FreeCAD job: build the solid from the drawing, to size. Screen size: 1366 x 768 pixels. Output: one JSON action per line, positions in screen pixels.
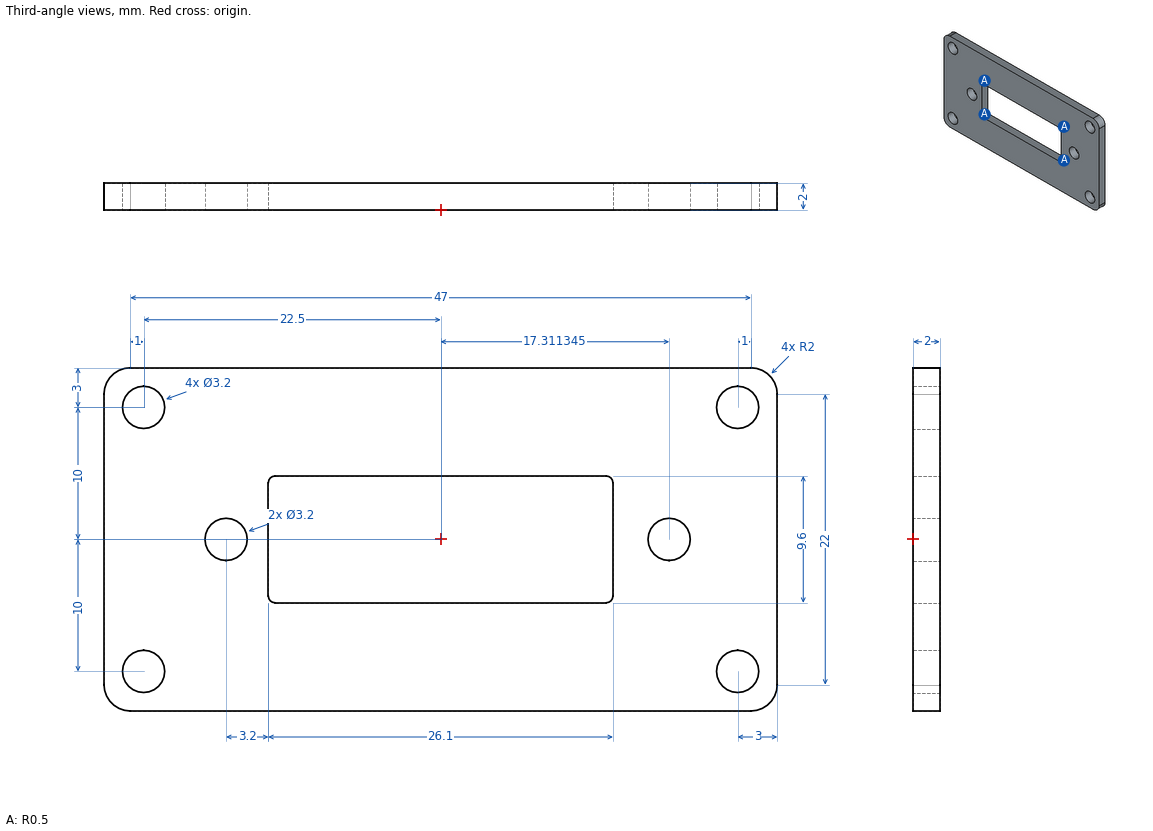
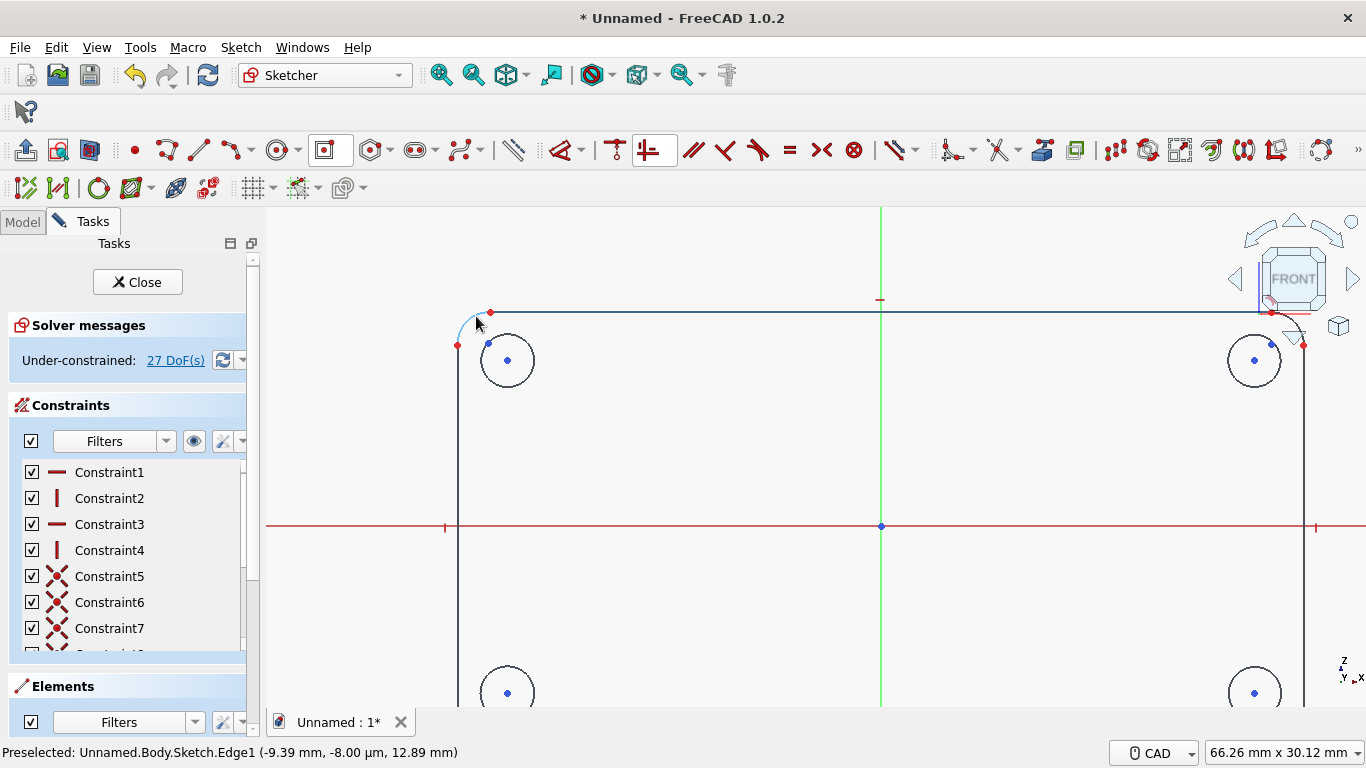
{"action": "left_click", "coordinate": [475, 315]}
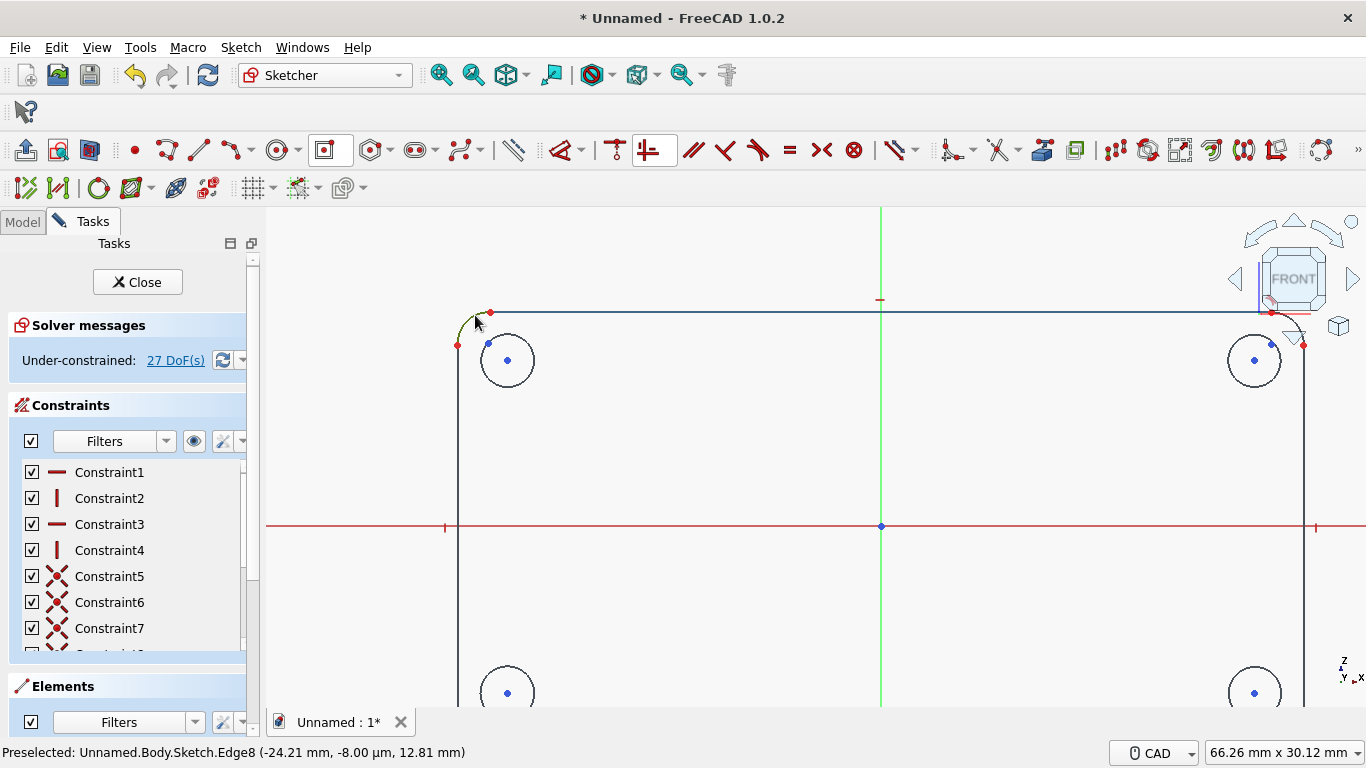
{"action": "left_click", "coordinate": [758, 150]}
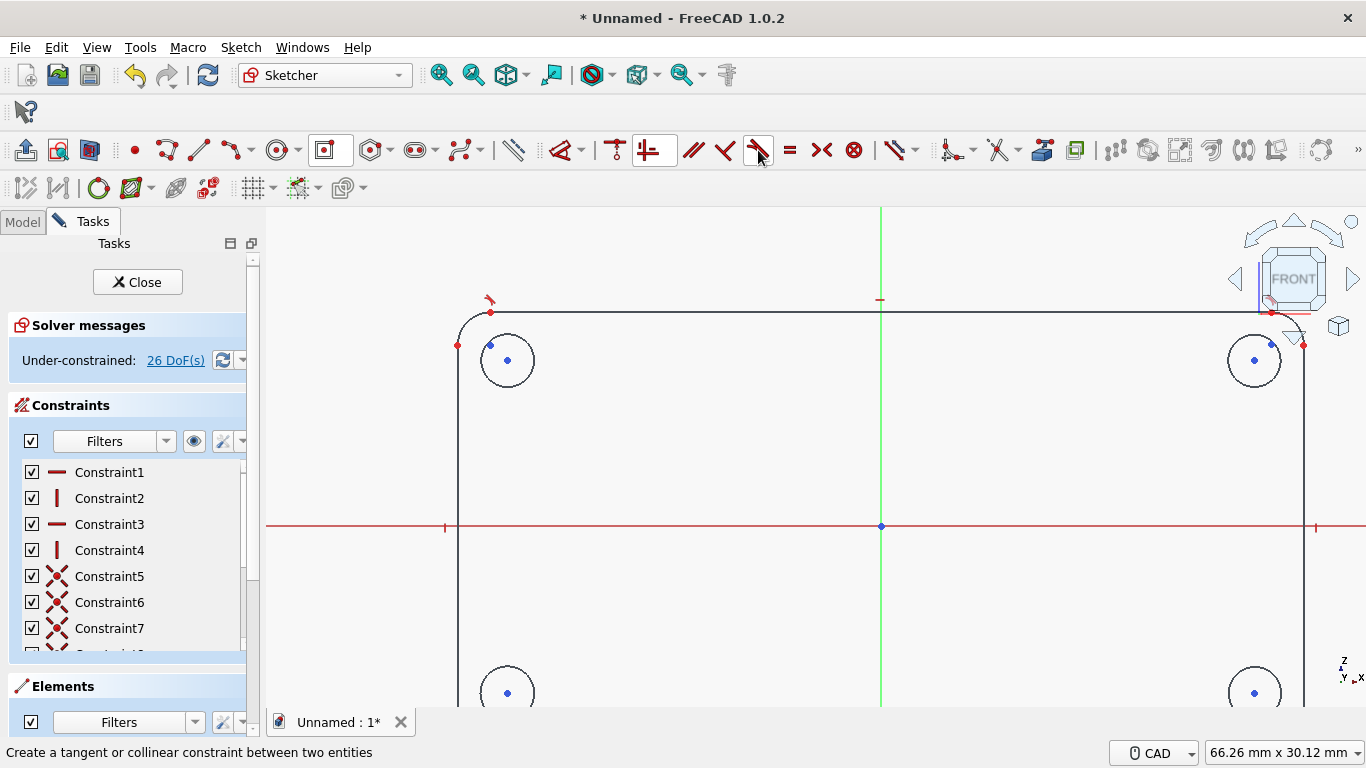
{"action": "scroll", "coordinate": [476, 316], "scroll_direction": "down", "scroll_amount": 2}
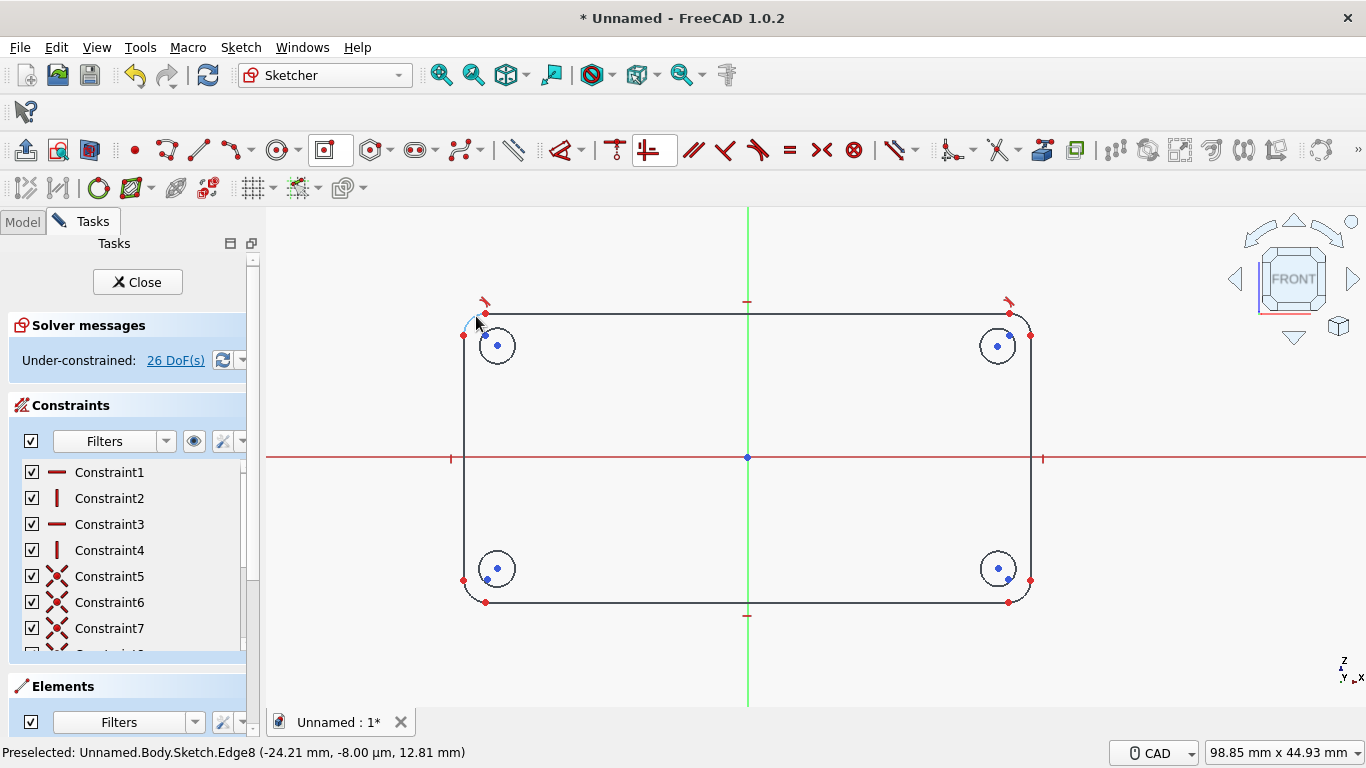
{"action": "left_click", "coordinate": [1031, 409]}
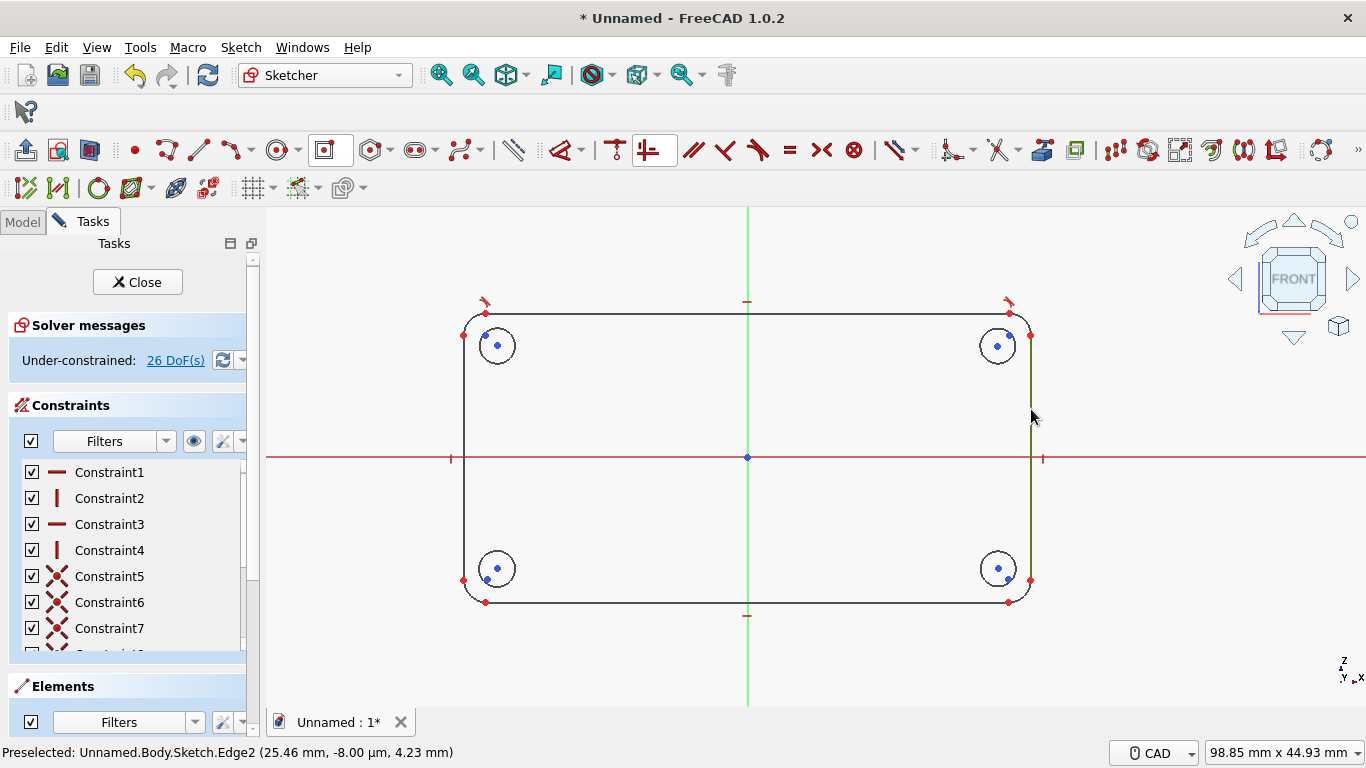
{"action": "scroll", "coordinate": [1029, 326], "scroll_direction": "up", "scroll_amount": 2}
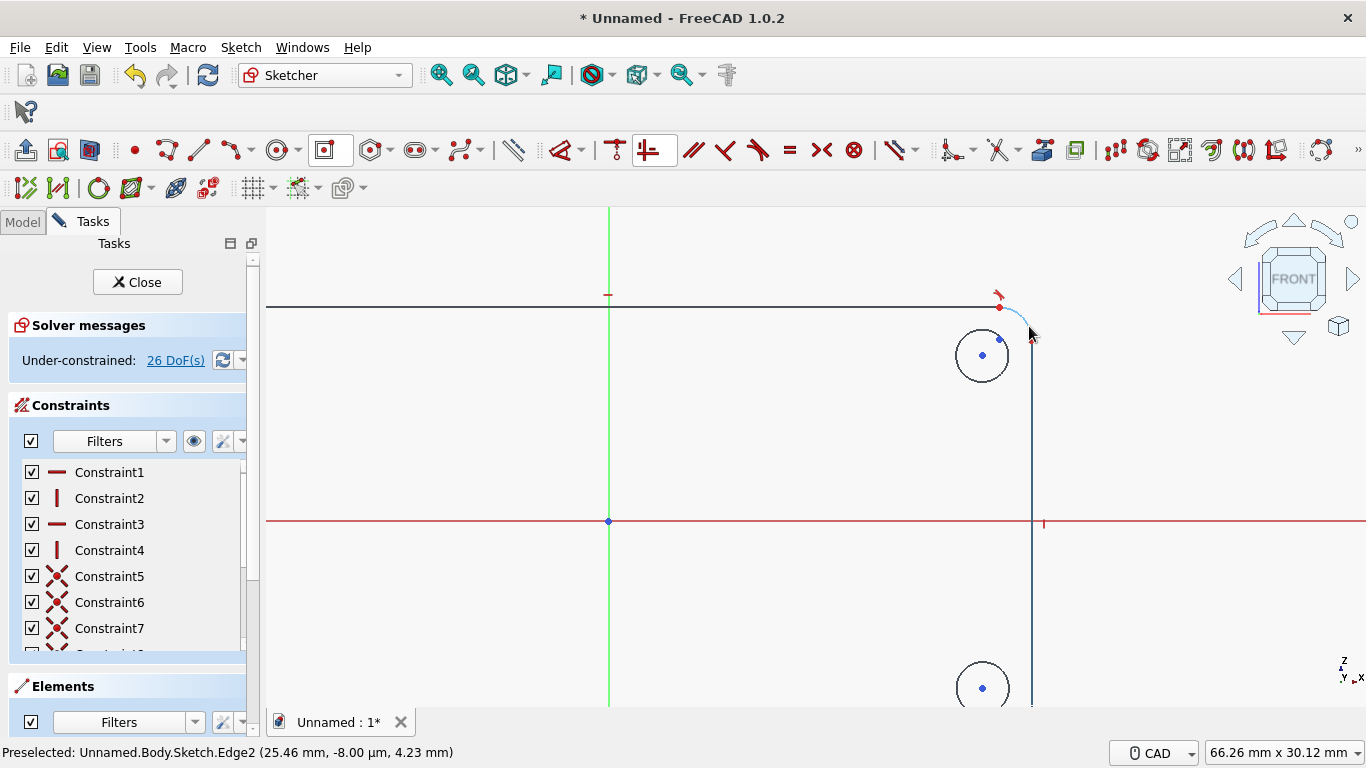
{"action": "left_click", "coordinate": [1028, 325]}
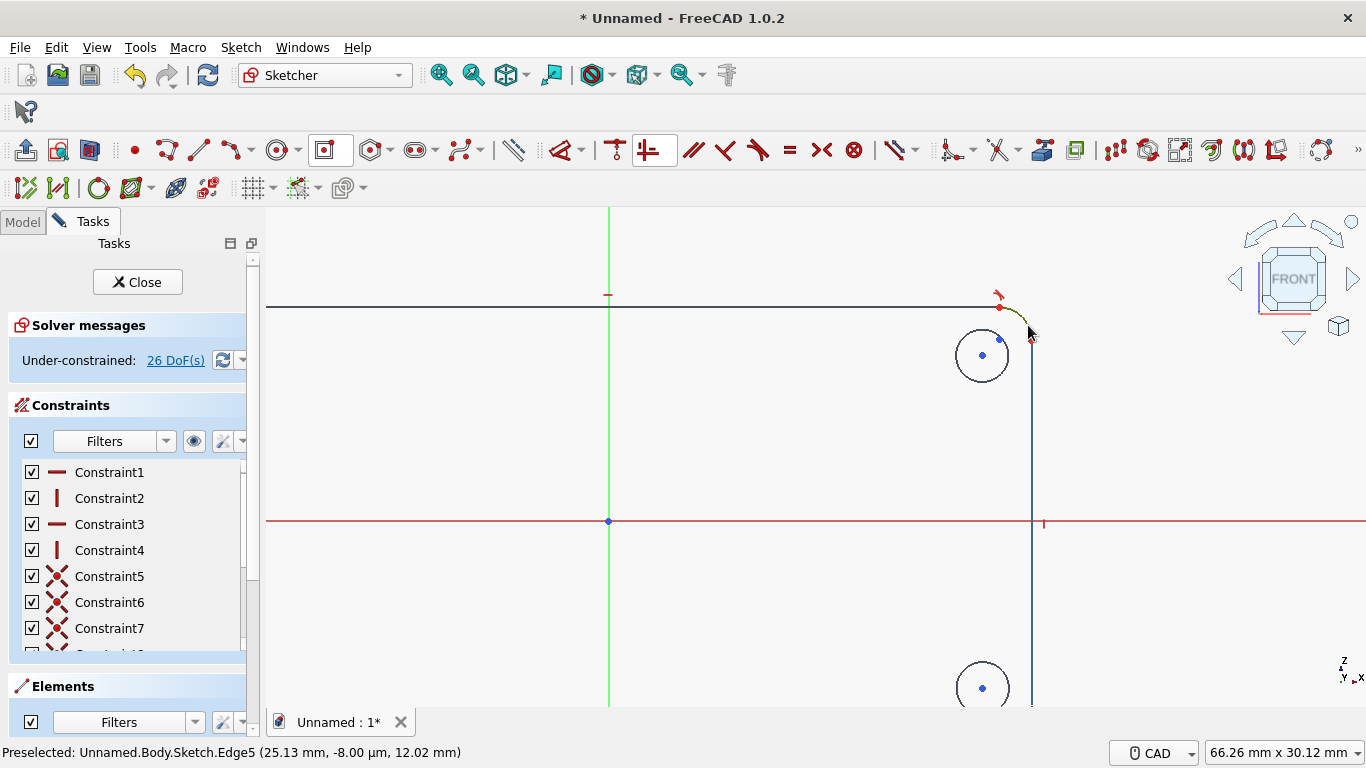
{"action": "left_click", "coordinate": [758, 150]}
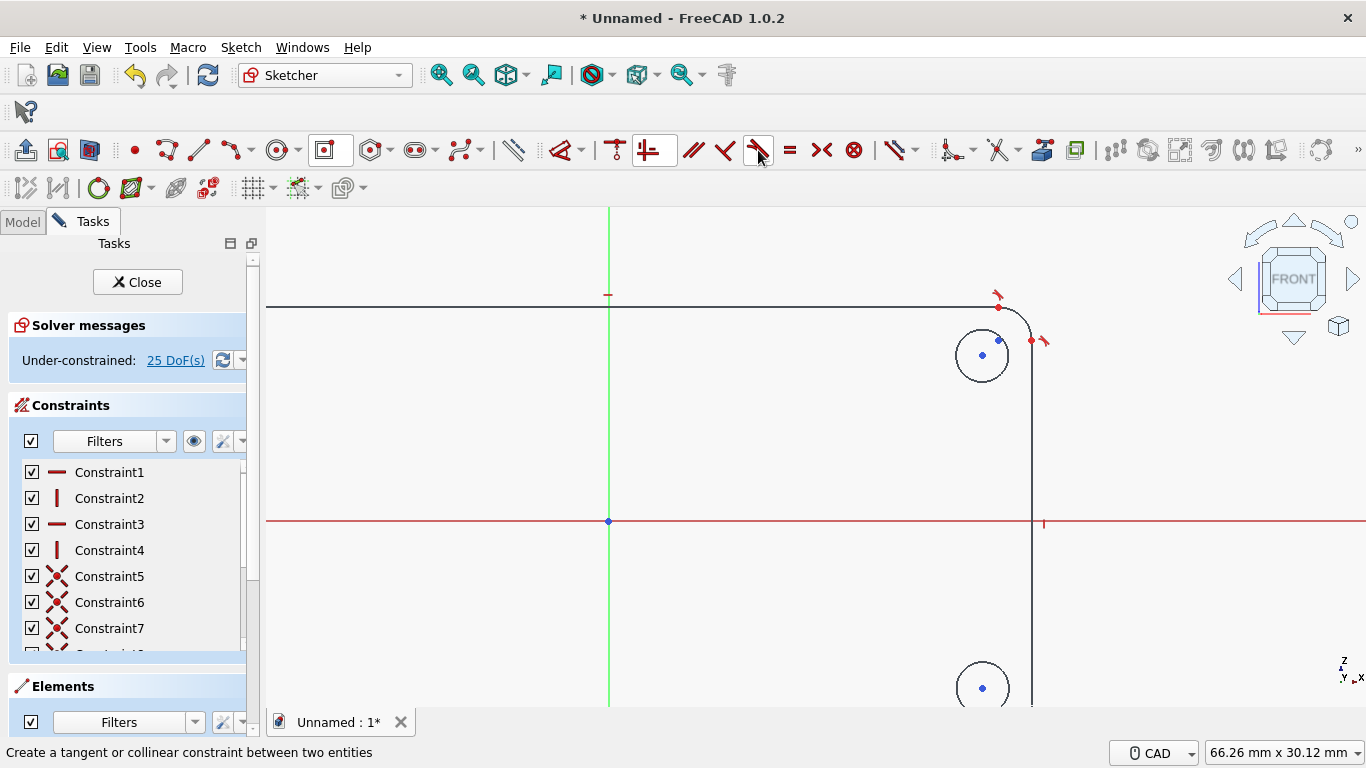
{"action": "left_click", "coordinate": [1032, 450]}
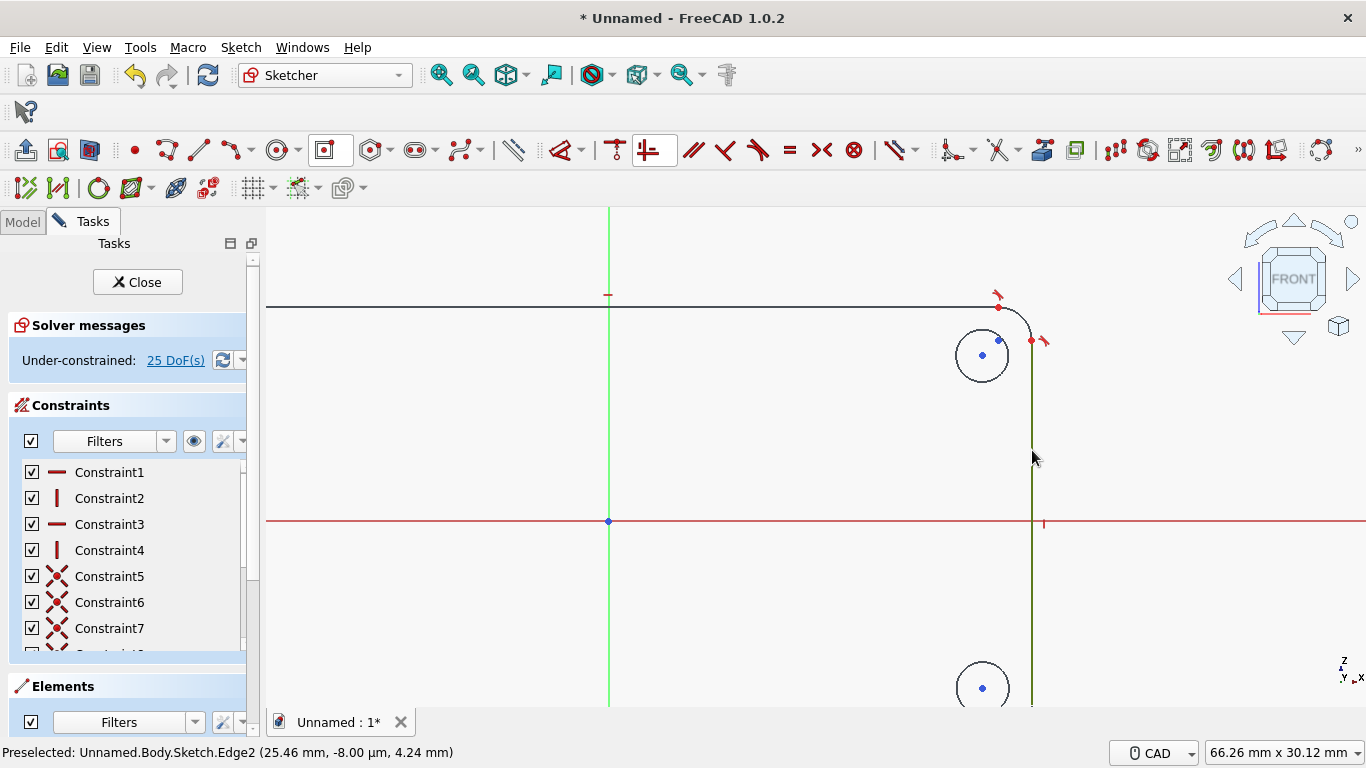
{"action": "scroll", "coordinate": [1029, 326], "scroll_direction": "down", "scroll_amount": 2}